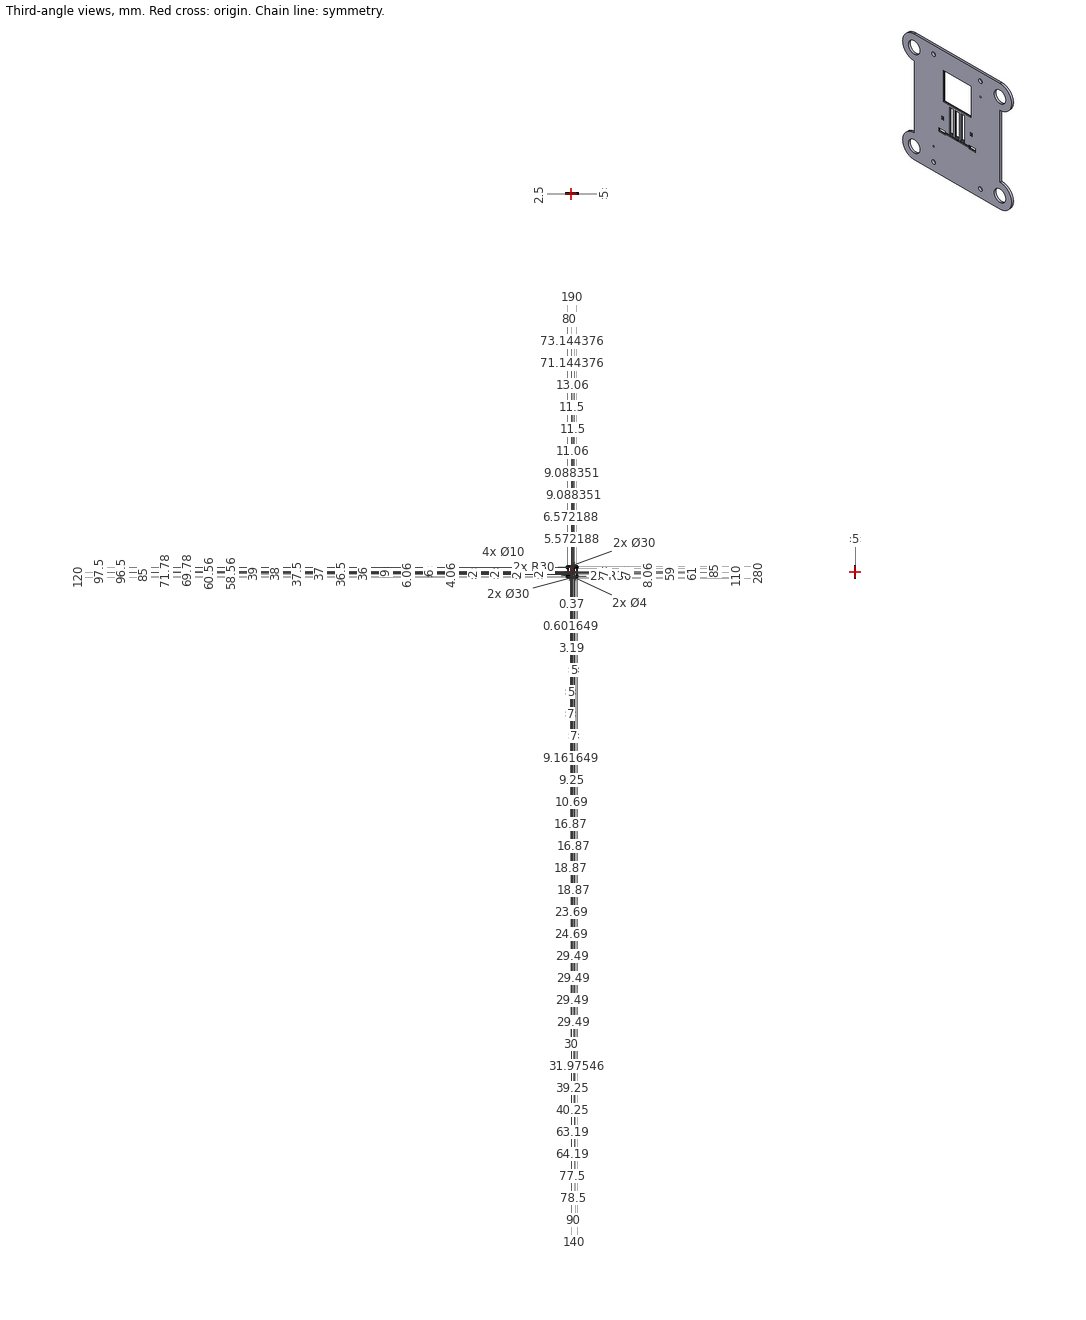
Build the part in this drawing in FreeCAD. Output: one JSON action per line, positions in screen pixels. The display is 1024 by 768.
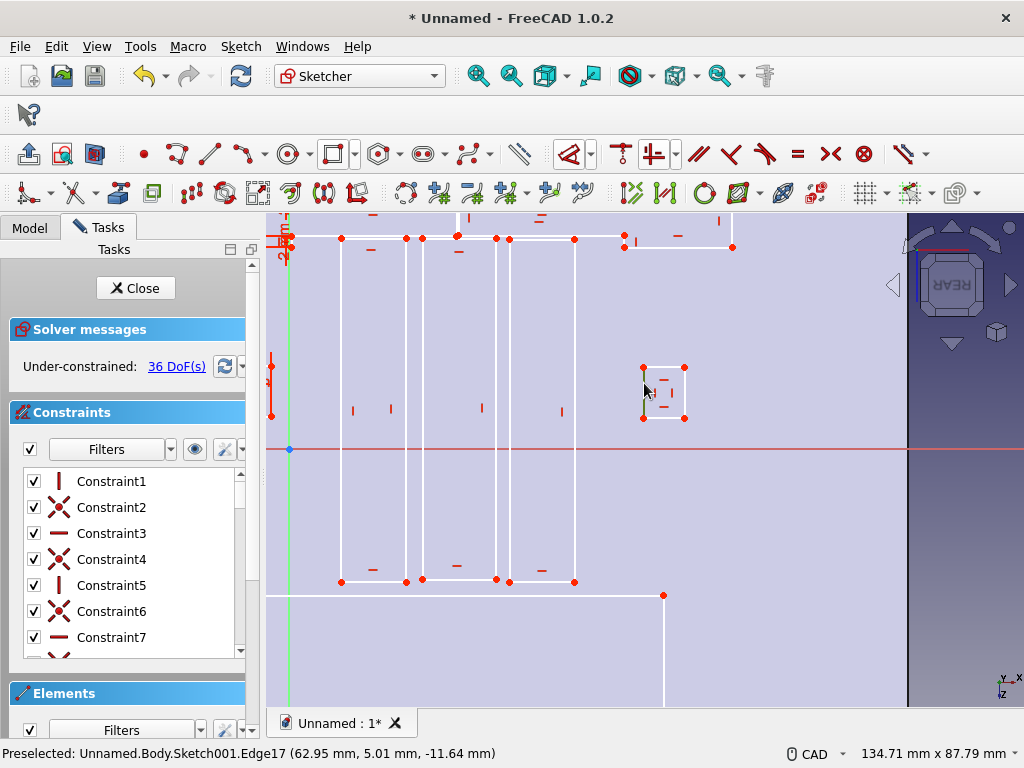
{"action": "key", "text": "i"}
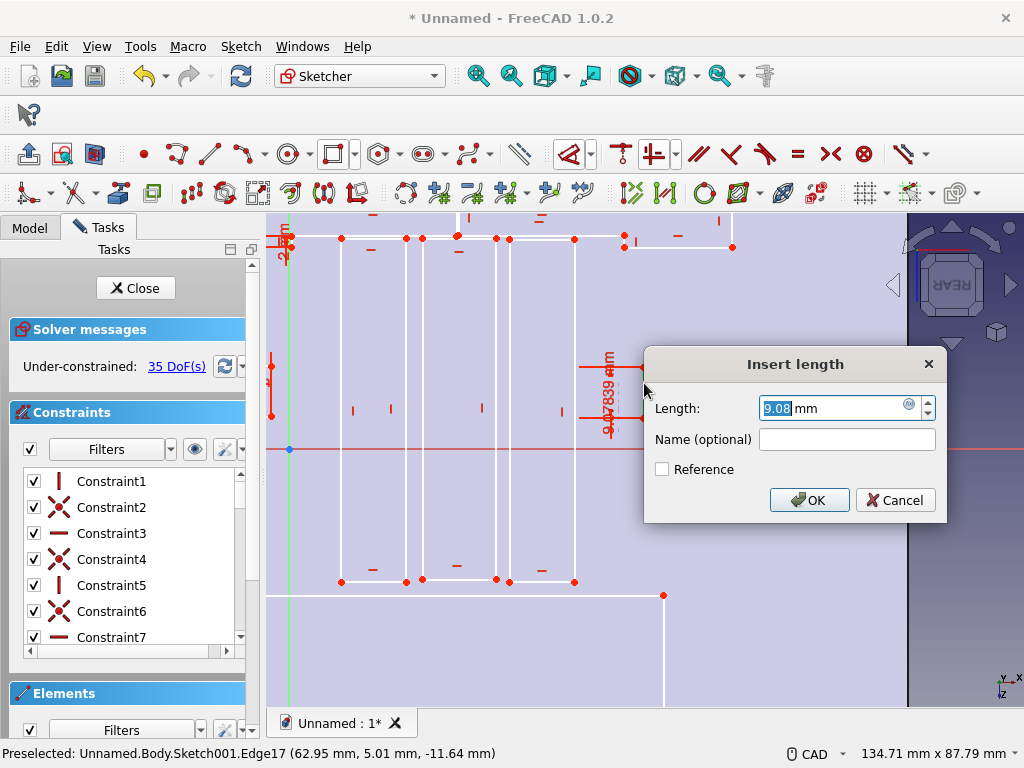
{"action": "type", "text": "9"}
{"action": "key", "text": "Return"}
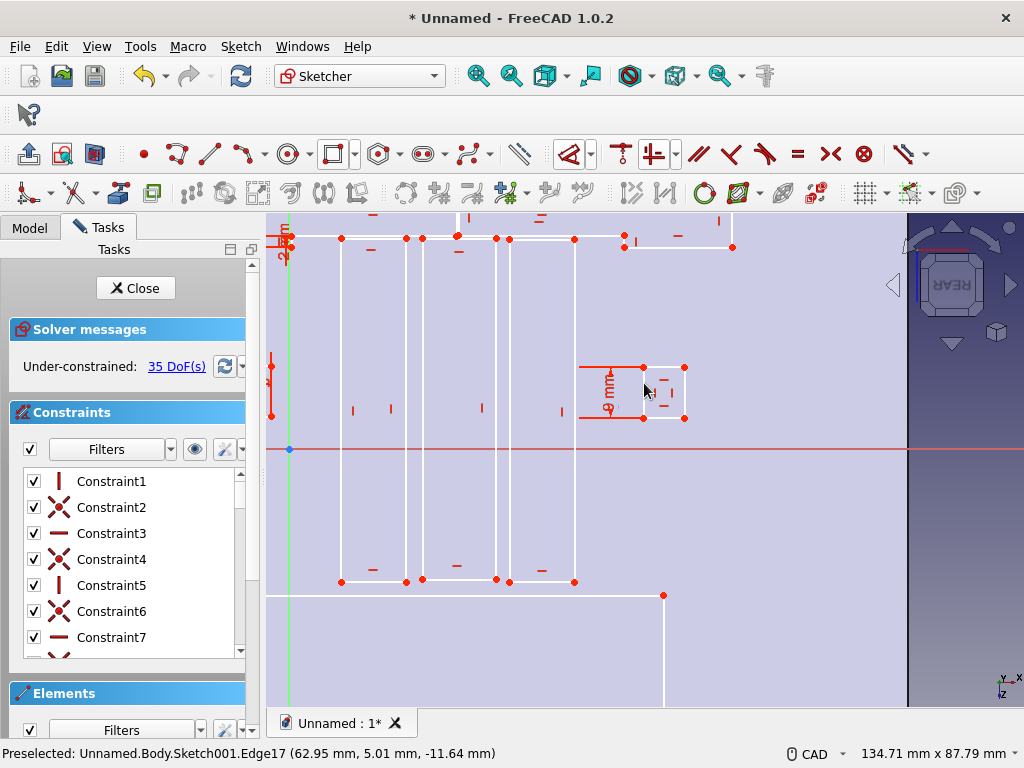
{"action": "left_click", "coordinate": [656, 418]}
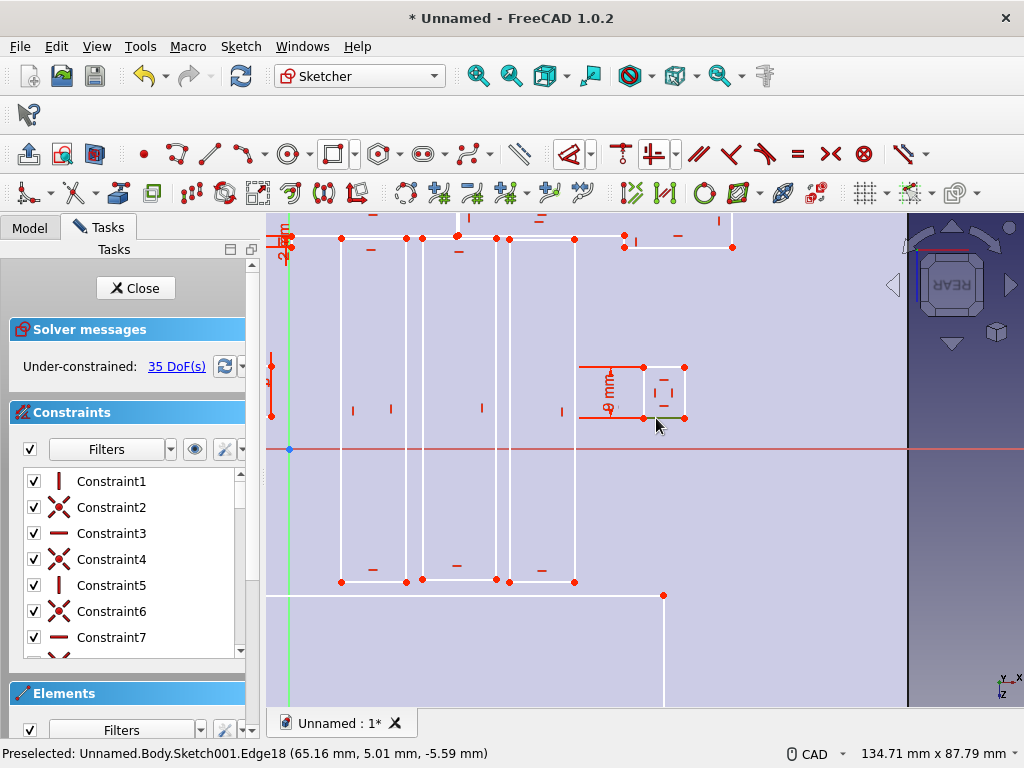
{"action": "left_click", "coordinate": [590, 154]}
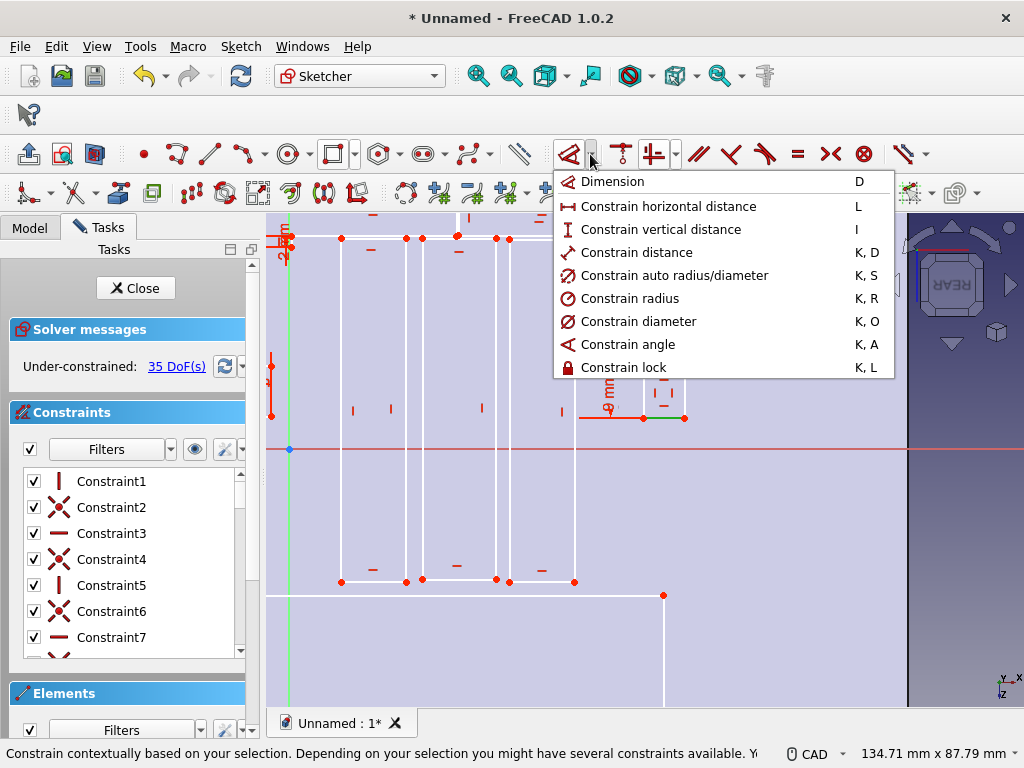
{"action": "left_click", "coordinate": [724, 206]}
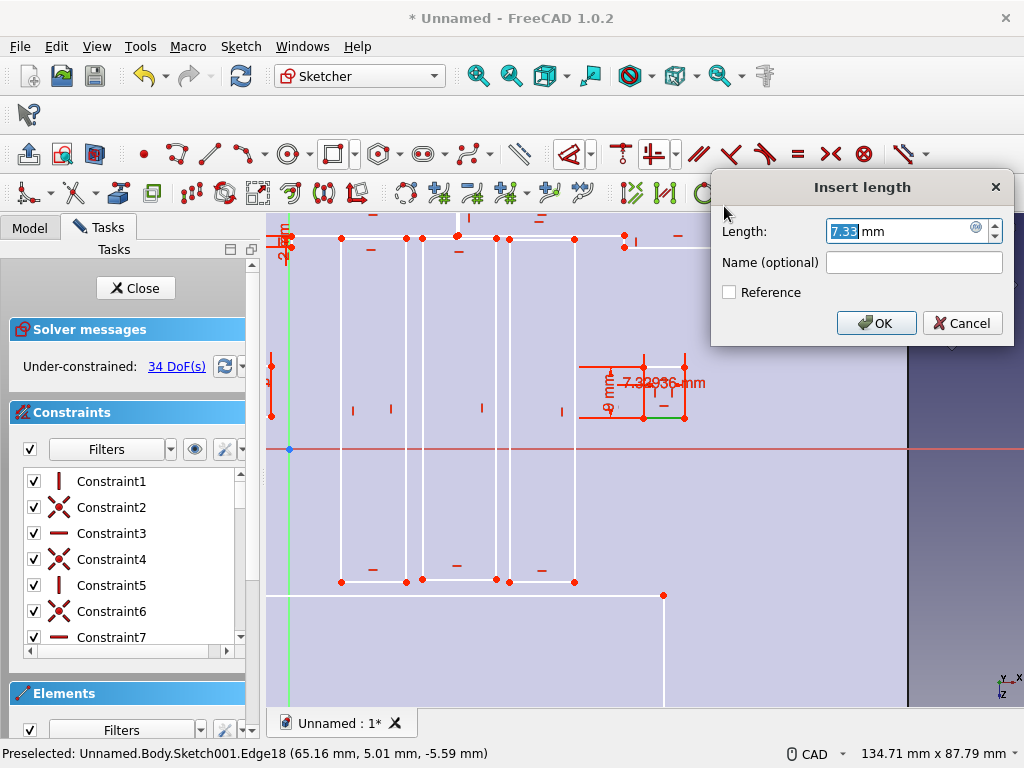
{"action": "type", "text": "7"}
{"action": "key", "text": "Return"}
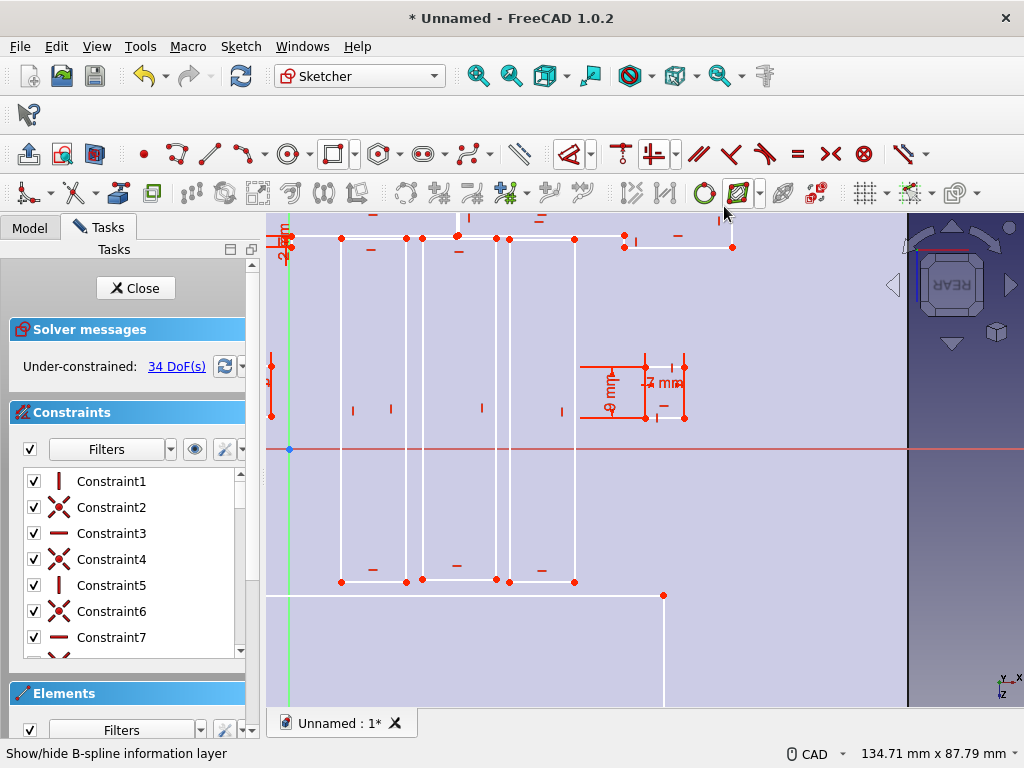
{"action": "scroll", "coordinate": [624, 242], "scroll_direction": "up", "scroll_amount": 7}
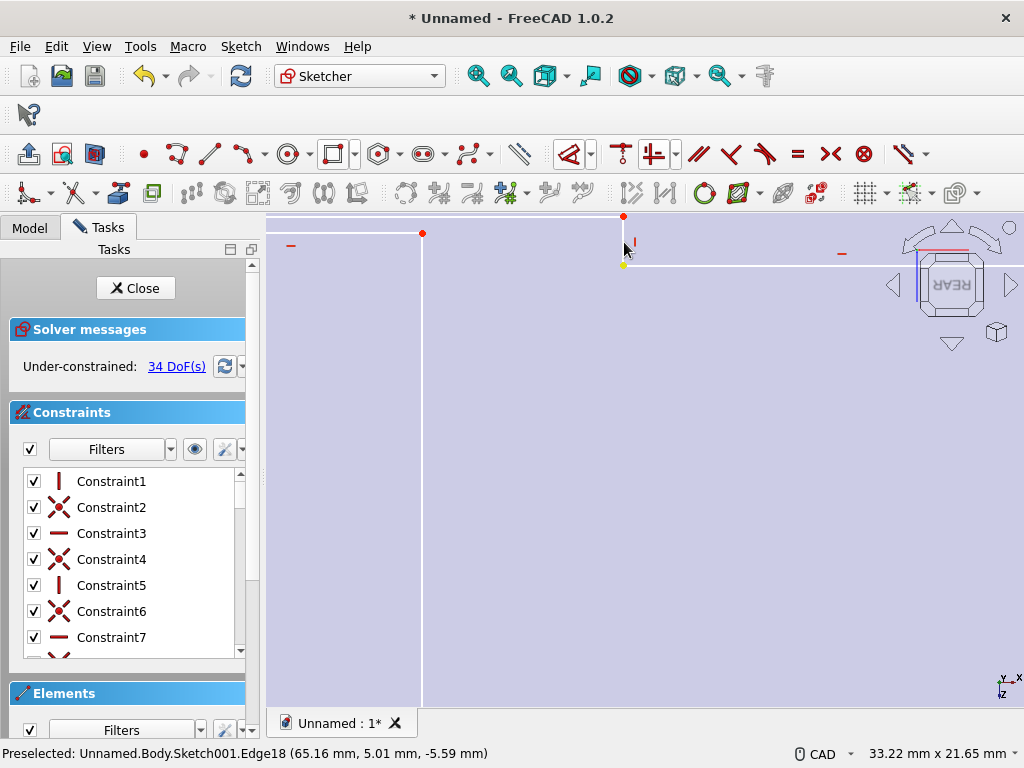
{"action": "left_click", "coordinate": [623, 241]}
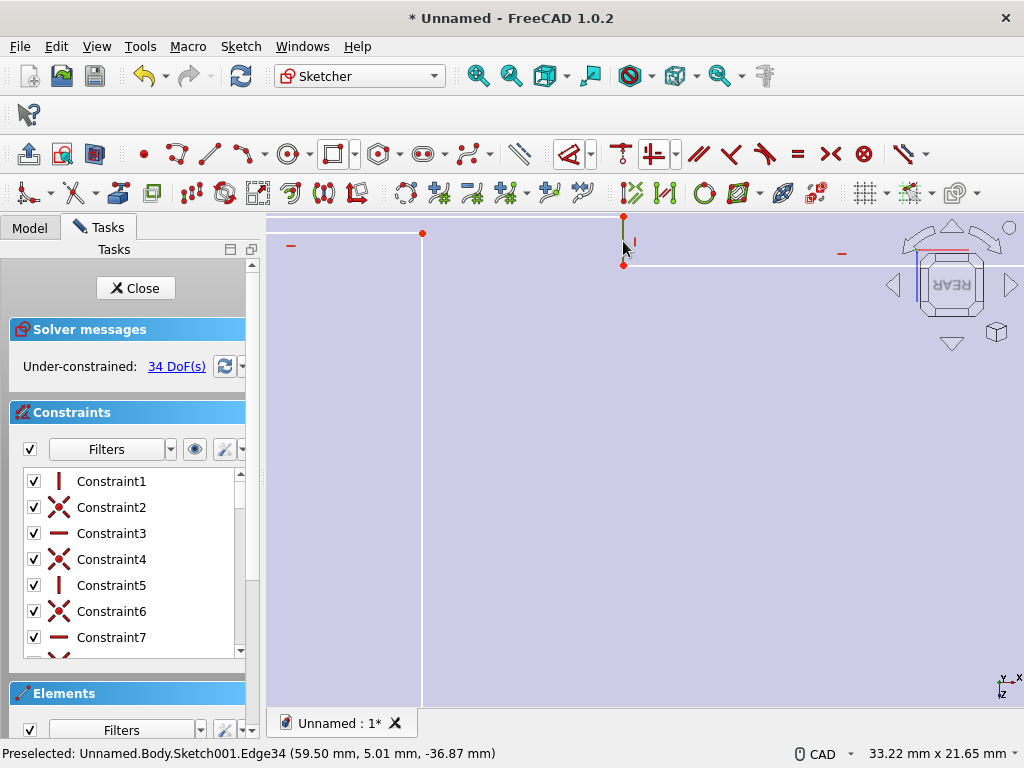
{"action": "key", "text": "i"}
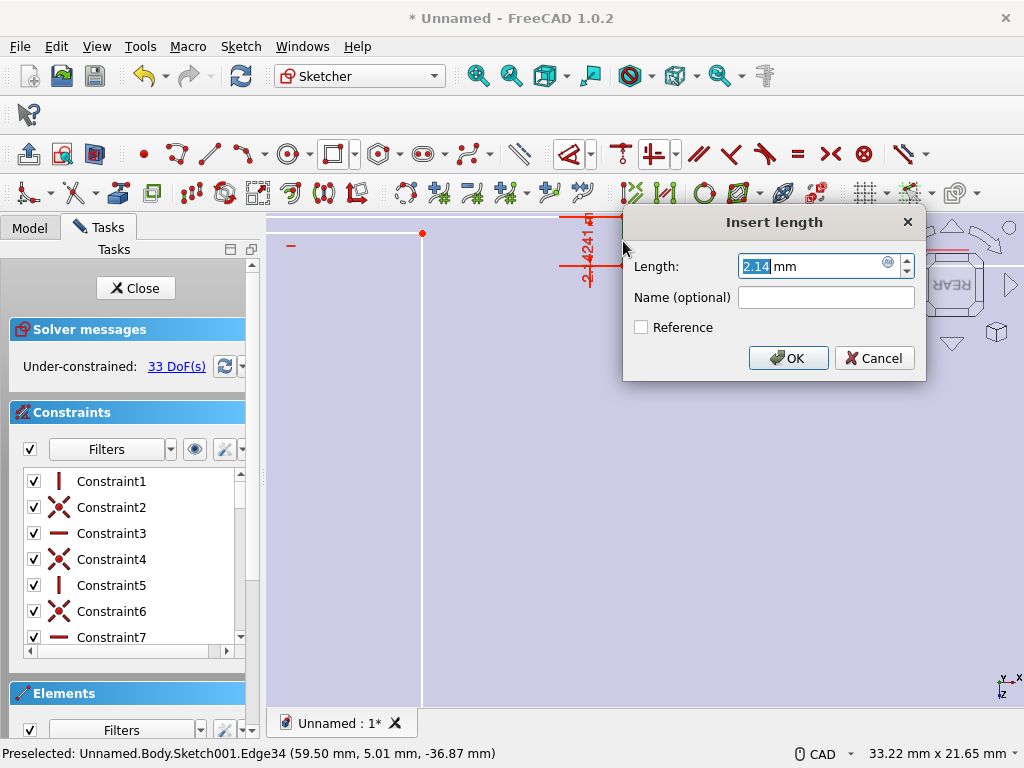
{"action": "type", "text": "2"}
{"action": "key", "text": "Return"}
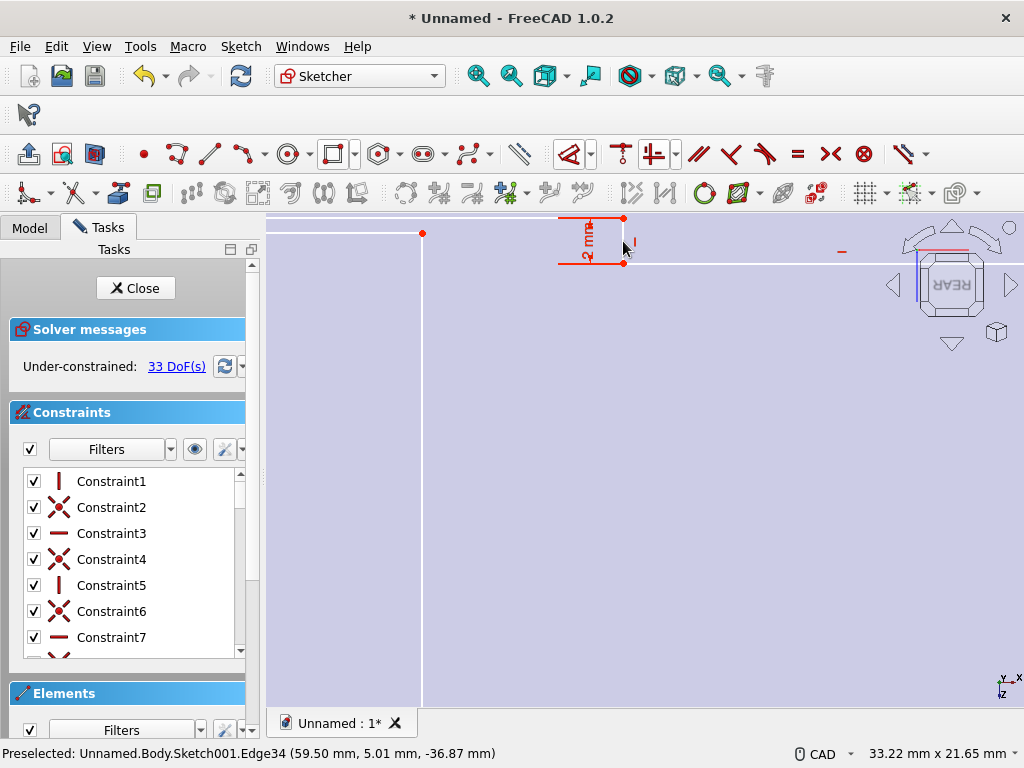
{"action": "scroll", "coordinate": [639, 339], "scroll_direction": "down", "scroll_amount": 12}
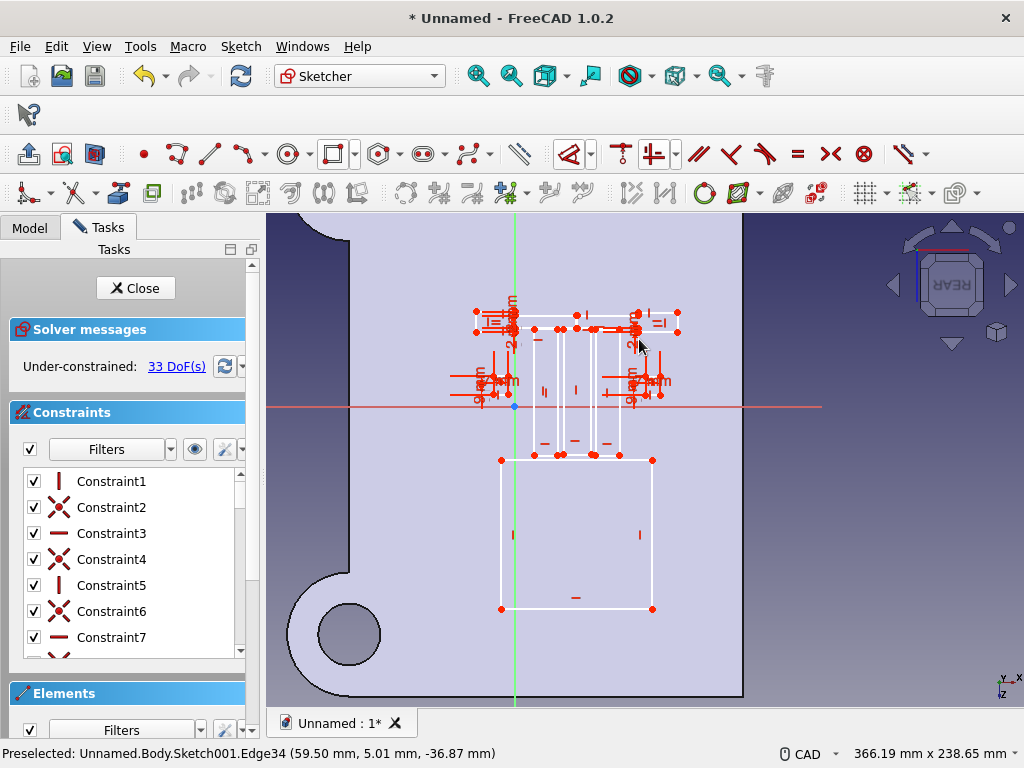
{"action": "scroll", "coordinate": [639, 314], "scroll_direction": "up", "scroll_amount": 14}